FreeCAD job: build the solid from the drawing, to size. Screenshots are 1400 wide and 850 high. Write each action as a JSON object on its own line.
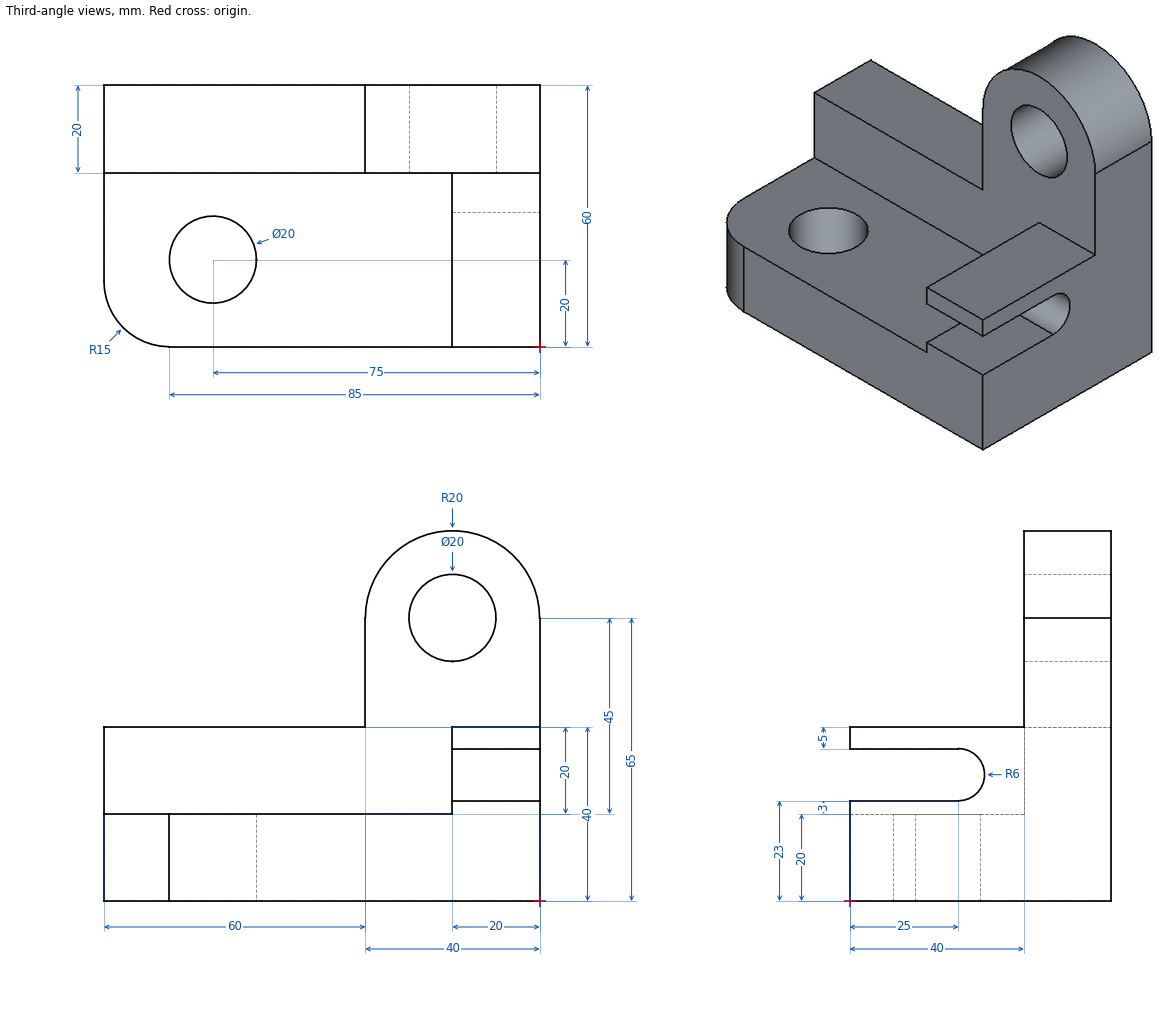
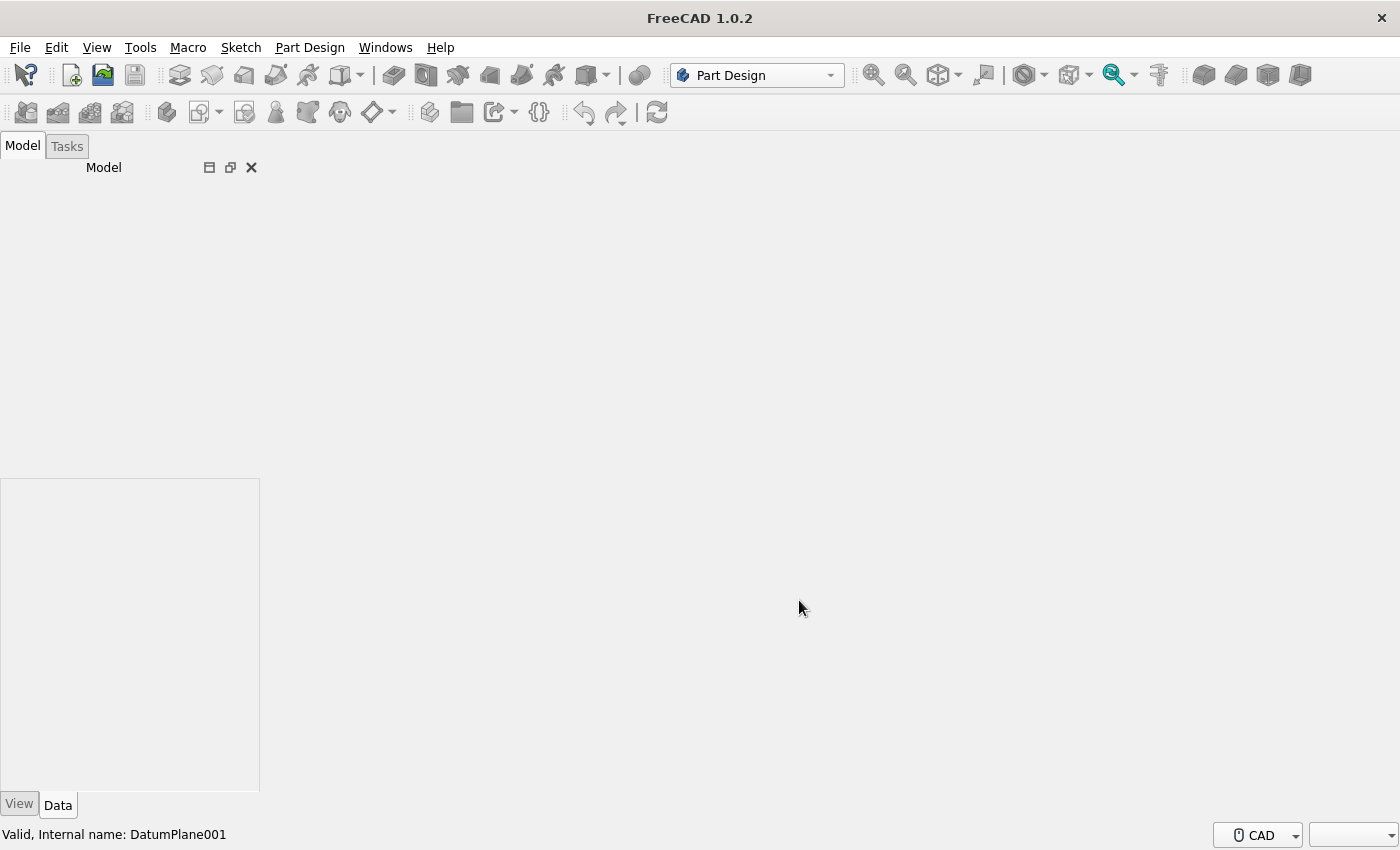
{"action": "left_click", "coordinate": [72, 76]}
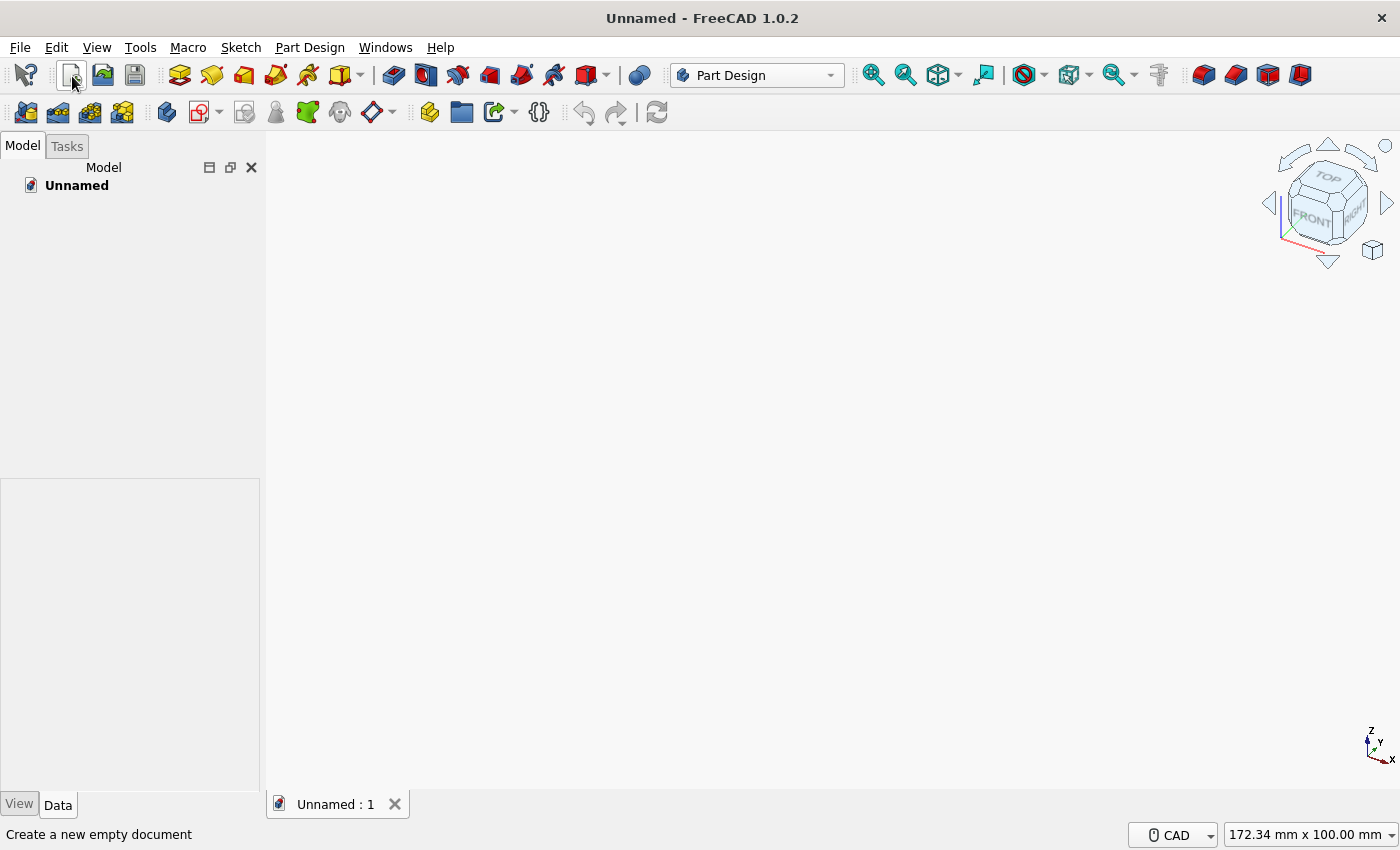
{"action": "left_click", "coordinate": [200, 112]}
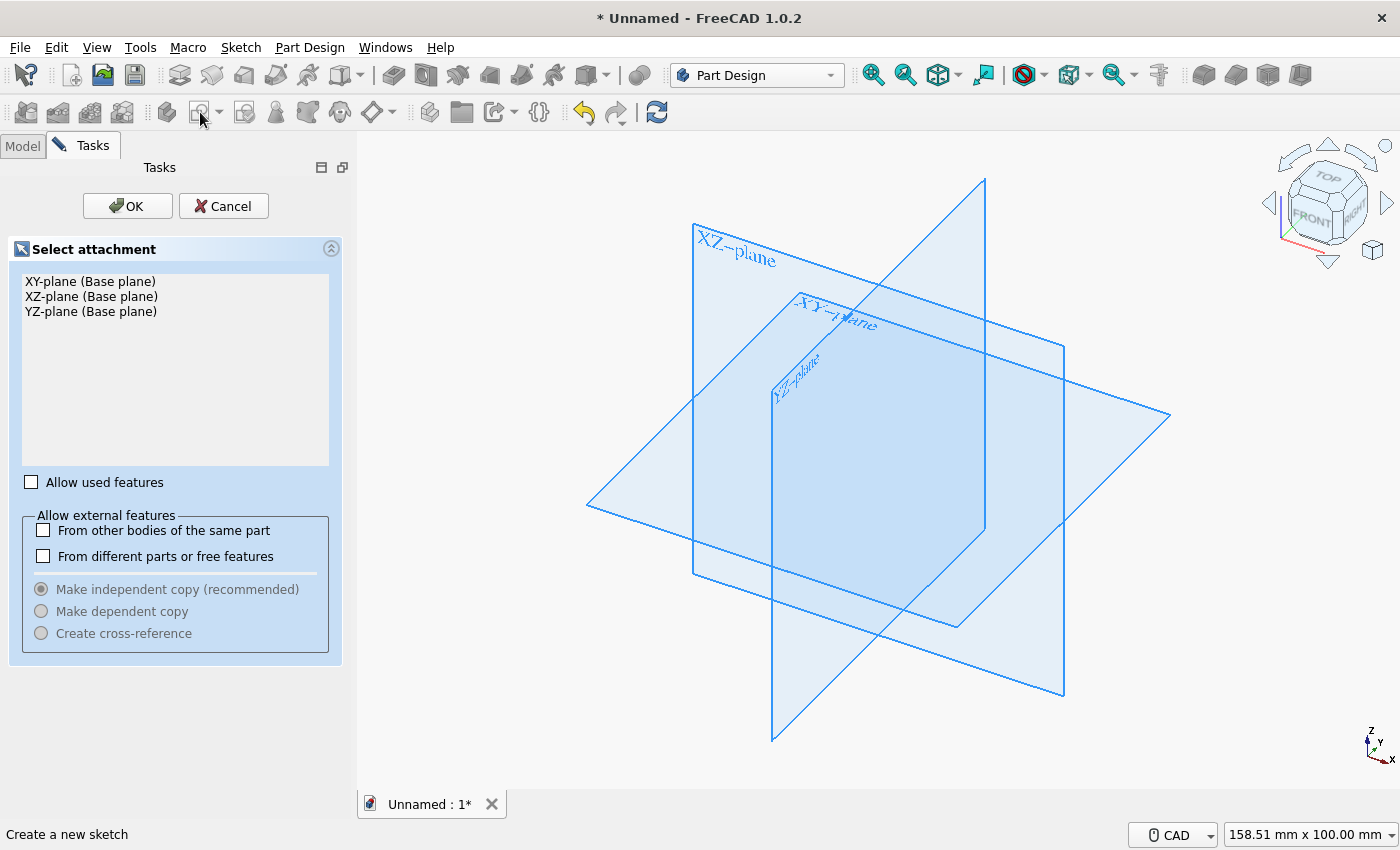
{"action": "left_click", "coordinate": [82, 282]}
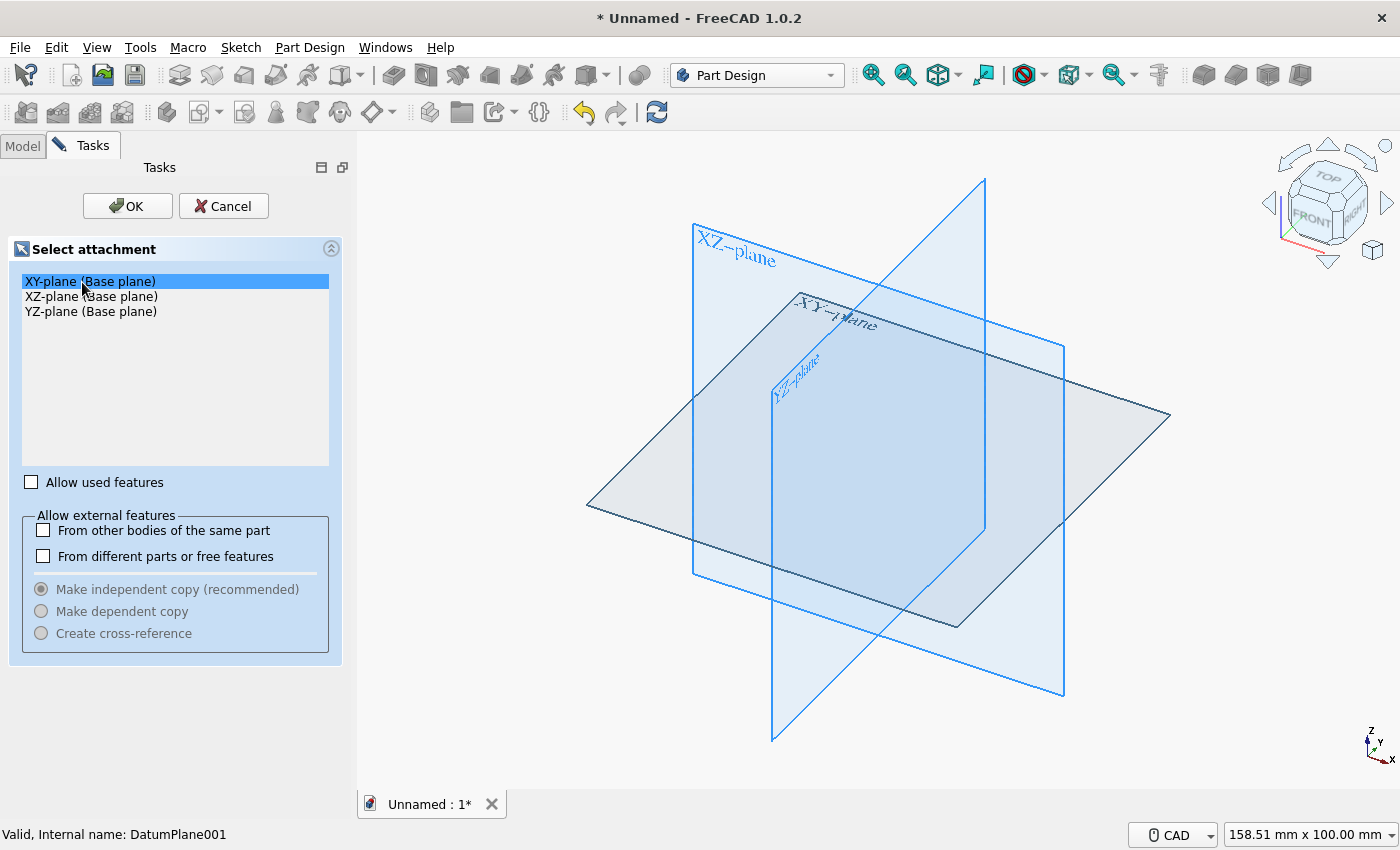
{"action": "left_click", "coordinate": [128, 206]}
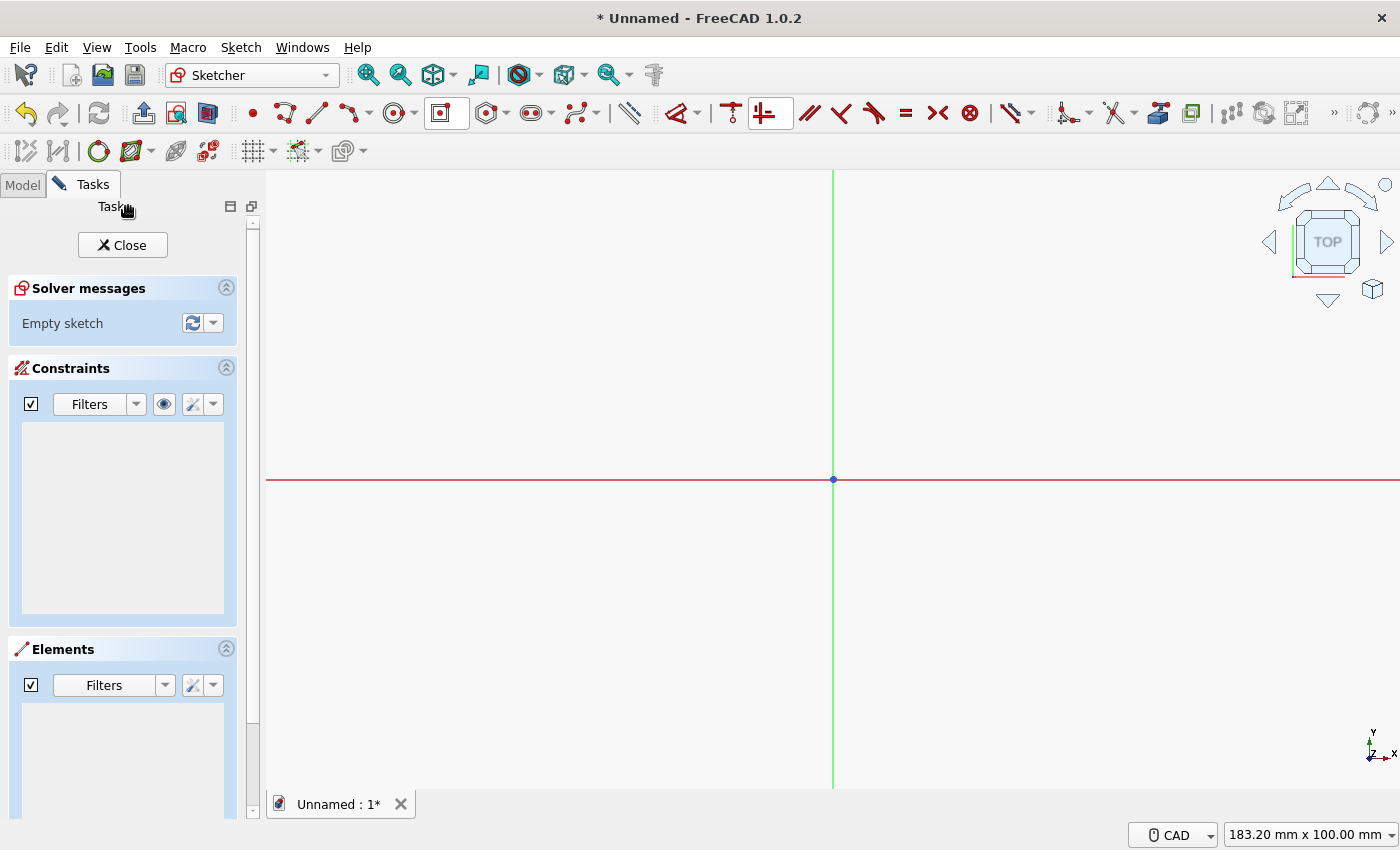
{"action": "scroll", "coordinate": [1235, 761], "scroll_direction": "down", "scroll_amount": 1}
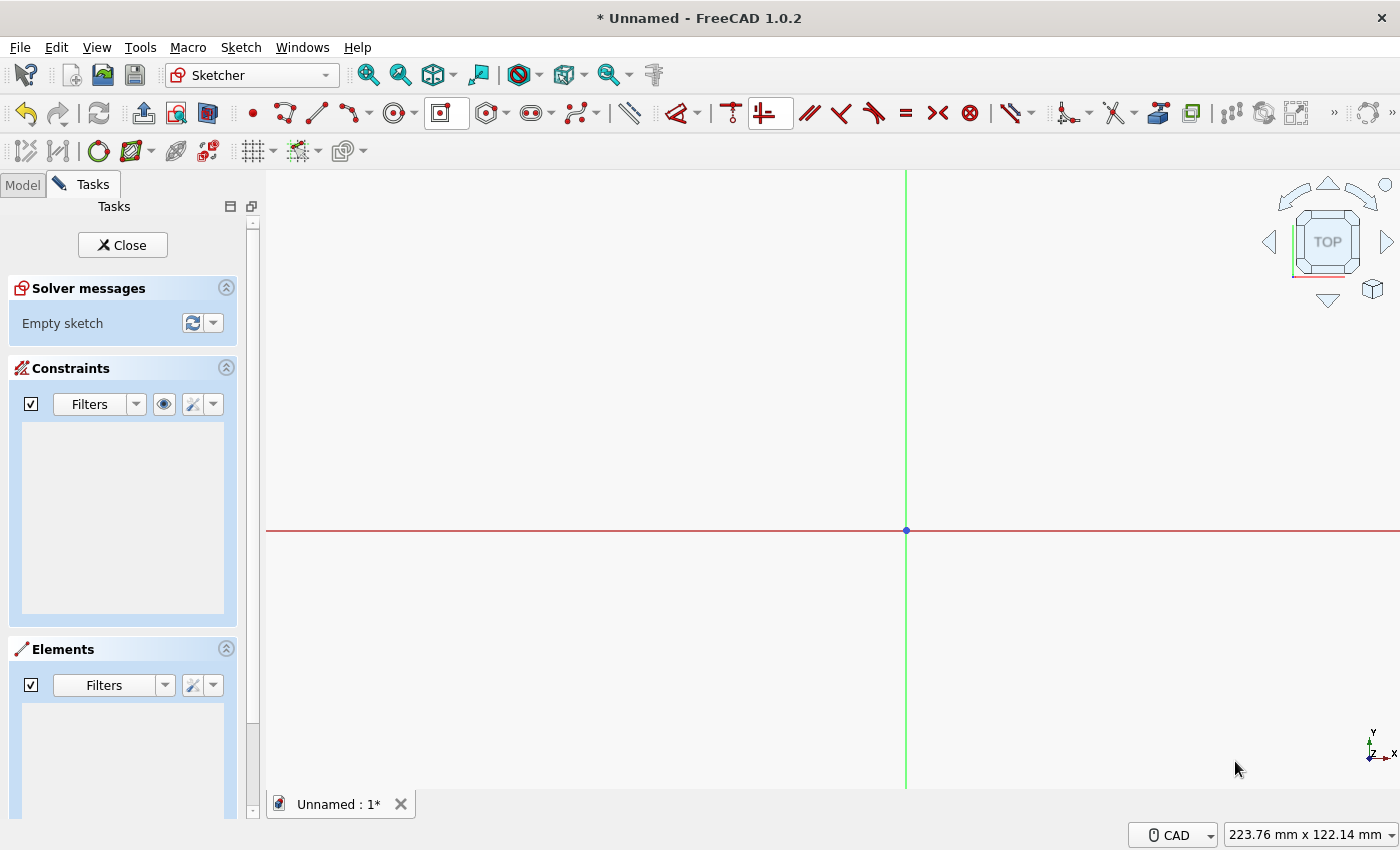
{"action": "key", "text": "g m"}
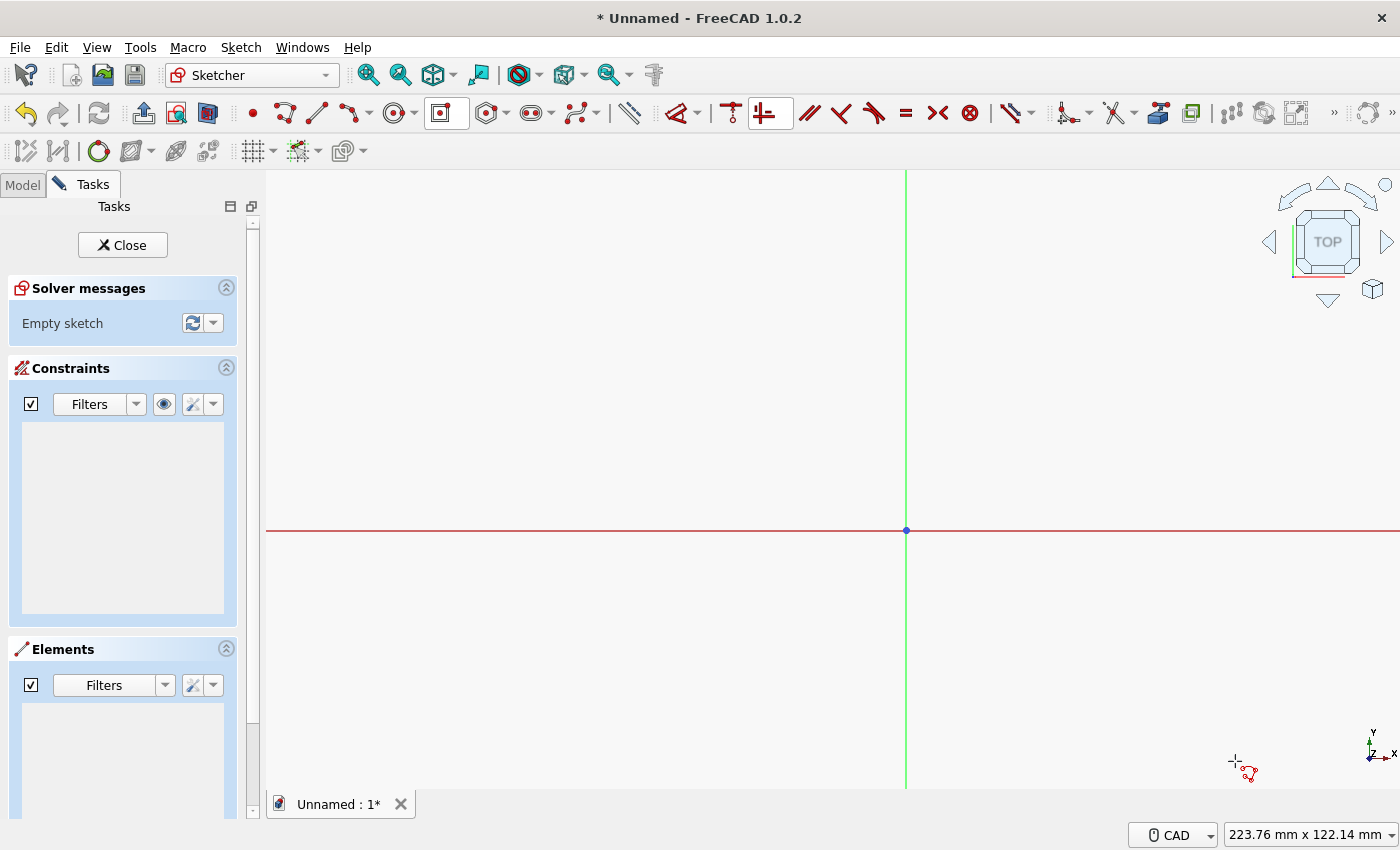
{"action": "left_click", "coordinate": [475, 531]}
{"action": "left_click", "coordinate": [906, 531]}
{"action": "left_click", "coordinate": [897, 227]}
{"action": "left_click", "coordinate": [399, 227]}
{"action": "left_click", "coordinate": [399, 455]}
{"action": "right_click", "coordinate": [399, 455]}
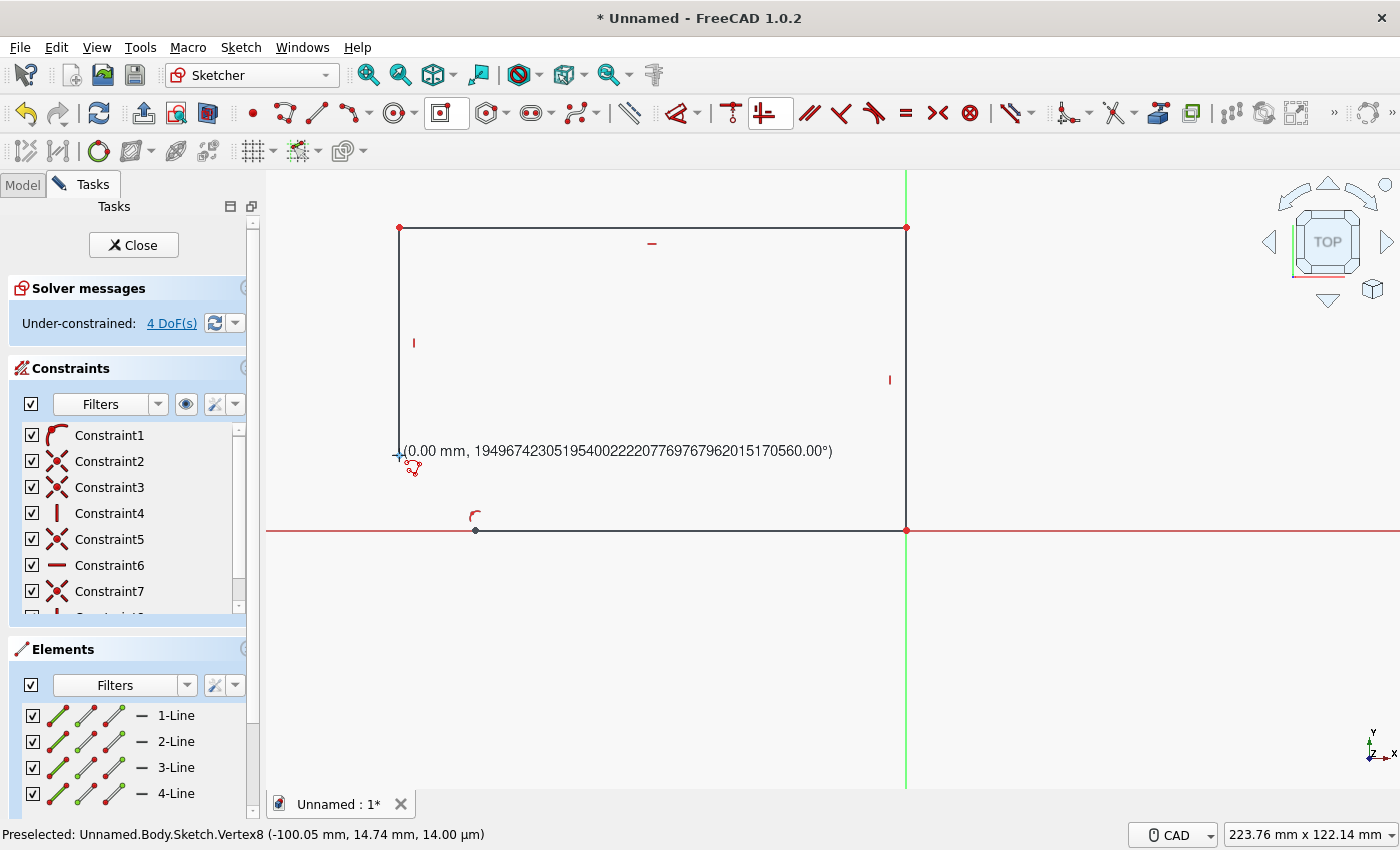
{"action": "key", "text": "g 3 a"}